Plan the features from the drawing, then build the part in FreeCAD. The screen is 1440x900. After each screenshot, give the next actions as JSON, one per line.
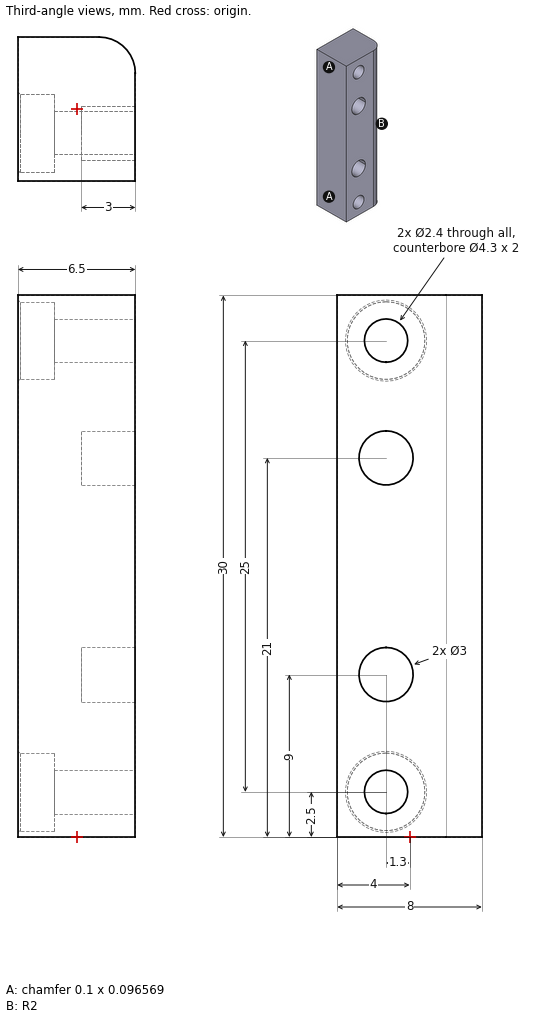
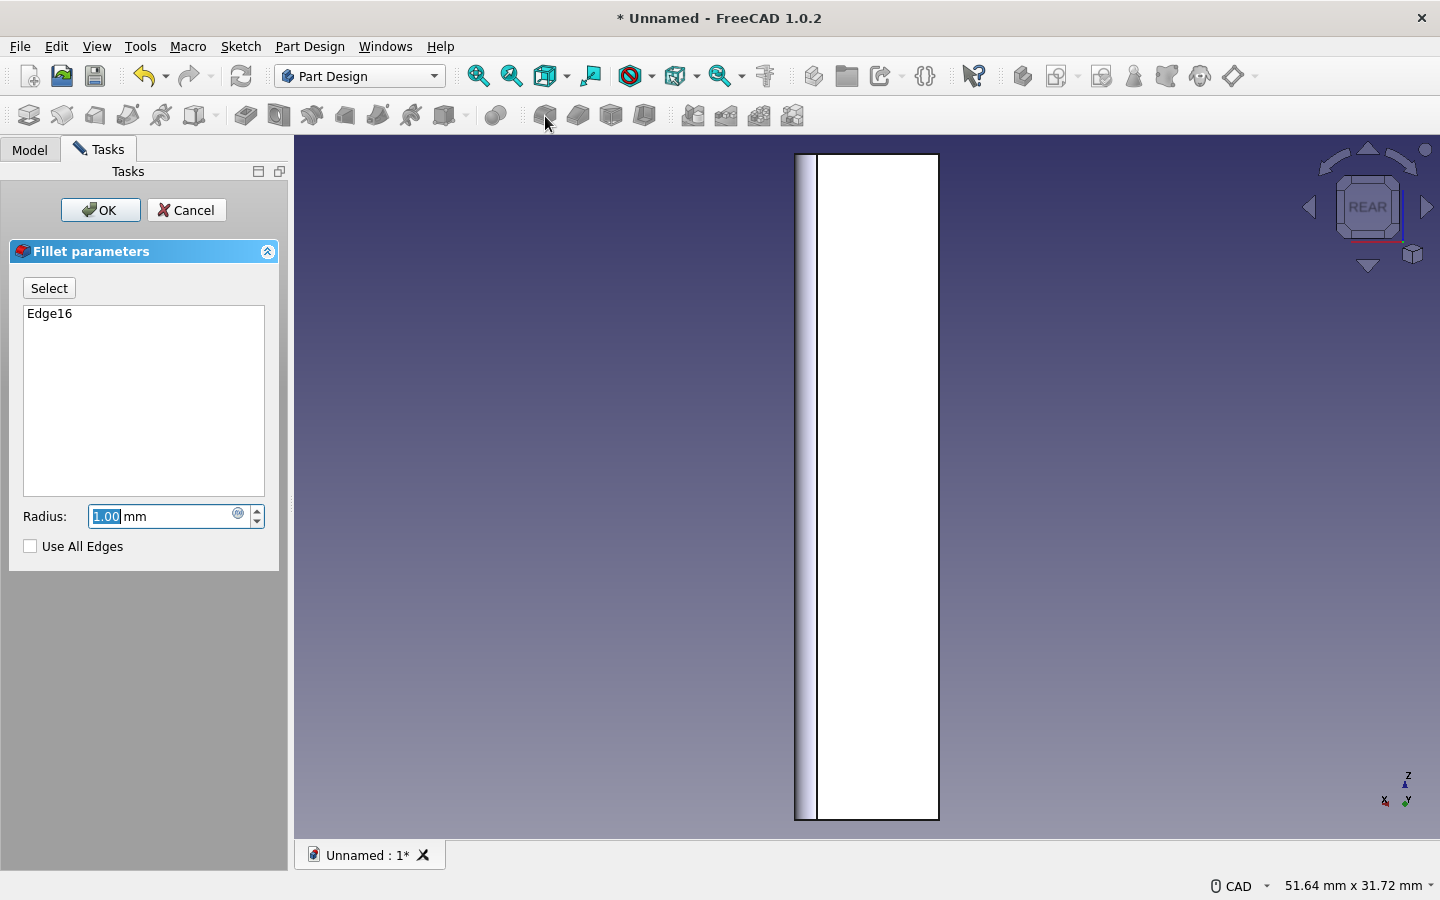
{"action": "type", "text": "2"}
{"action": "key", "text": "Tab"}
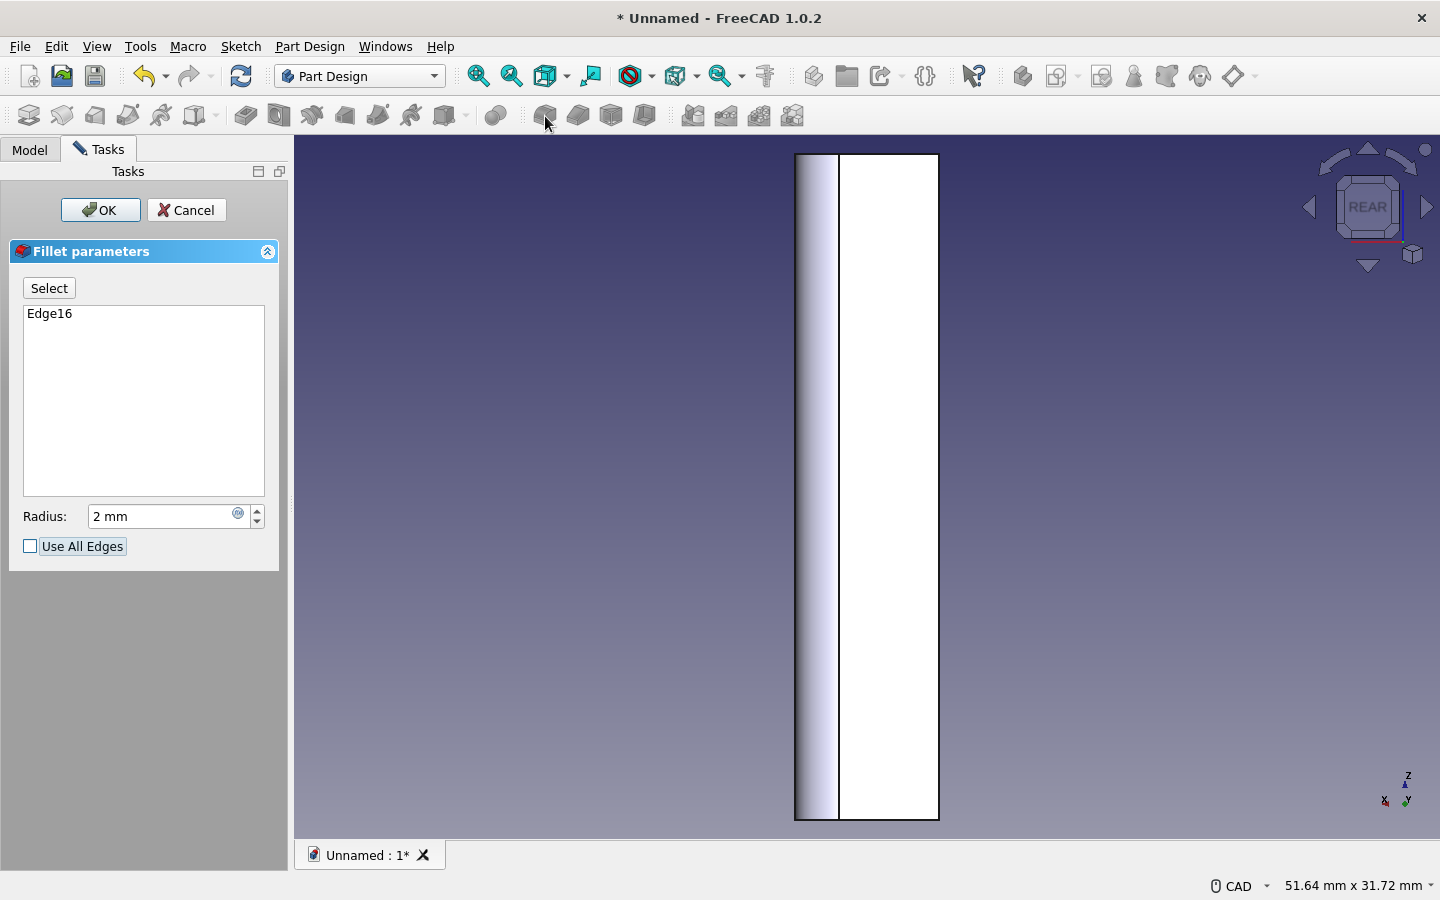
{"action": "left_click", "coordinate": [101, 210]}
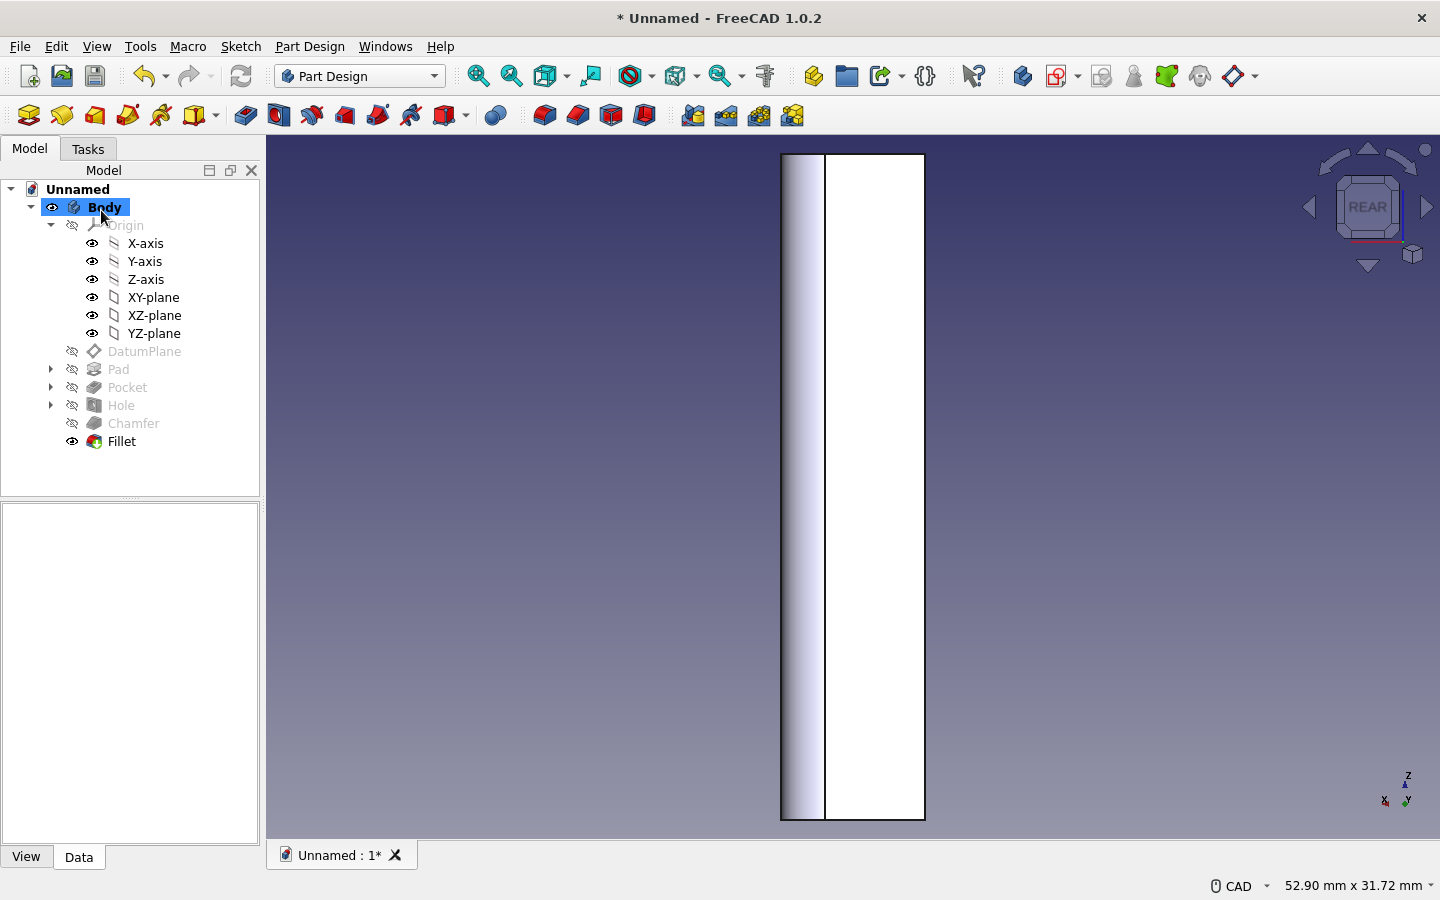
{"action": "key", "text": "0"}